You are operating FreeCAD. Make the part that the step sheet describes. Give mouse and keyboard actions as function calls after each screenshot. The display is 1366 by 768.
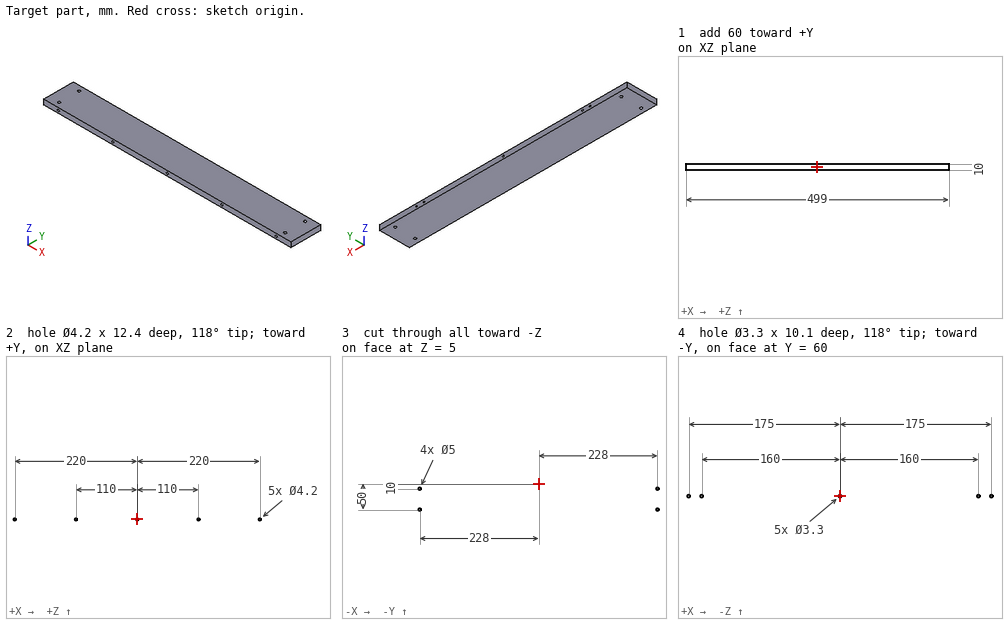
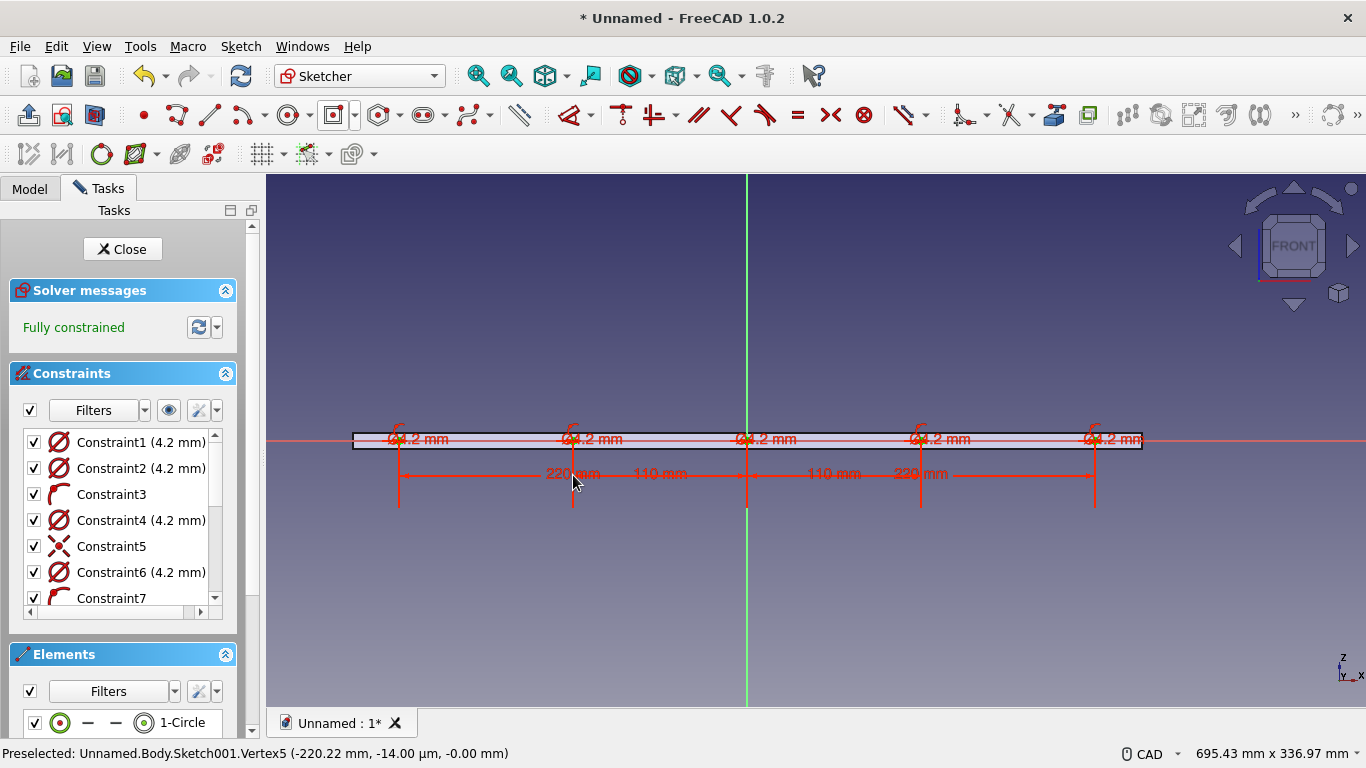
click(123, 249)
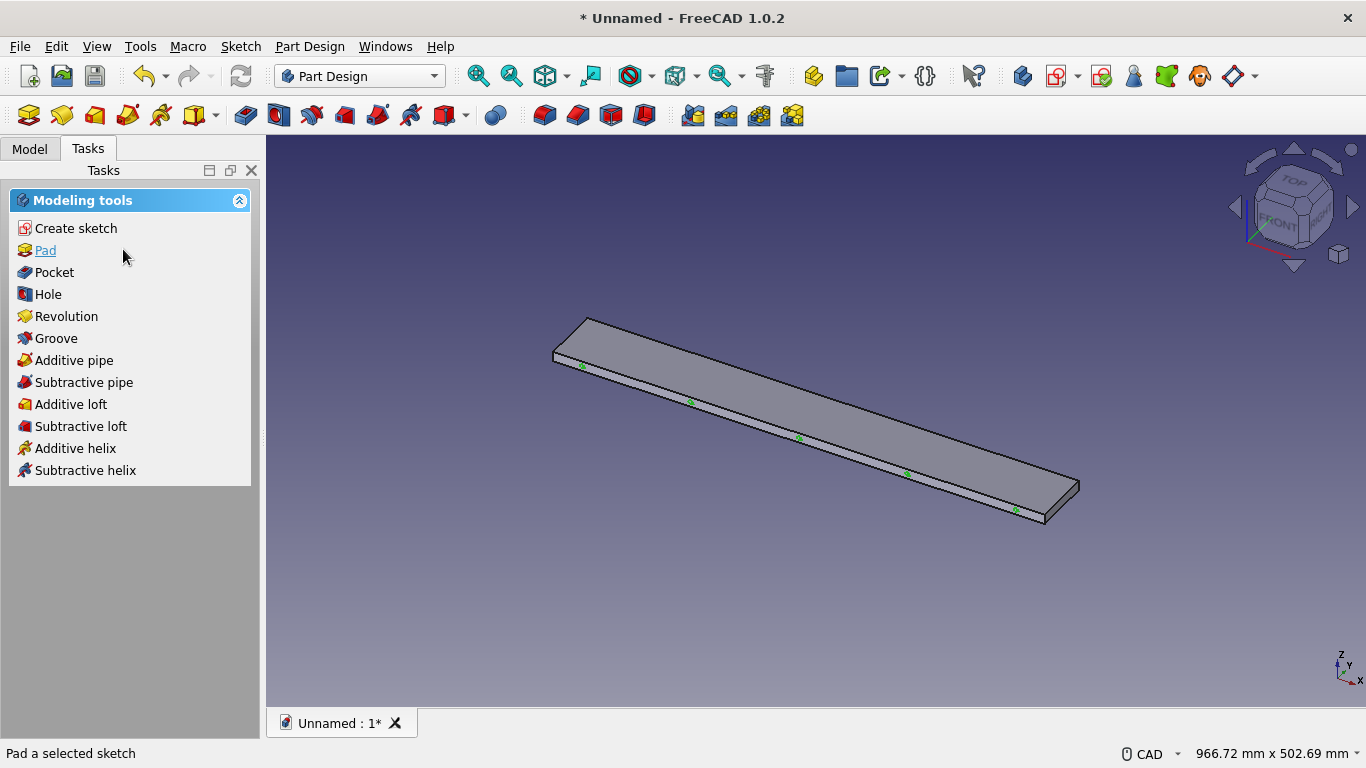
click(279, 116)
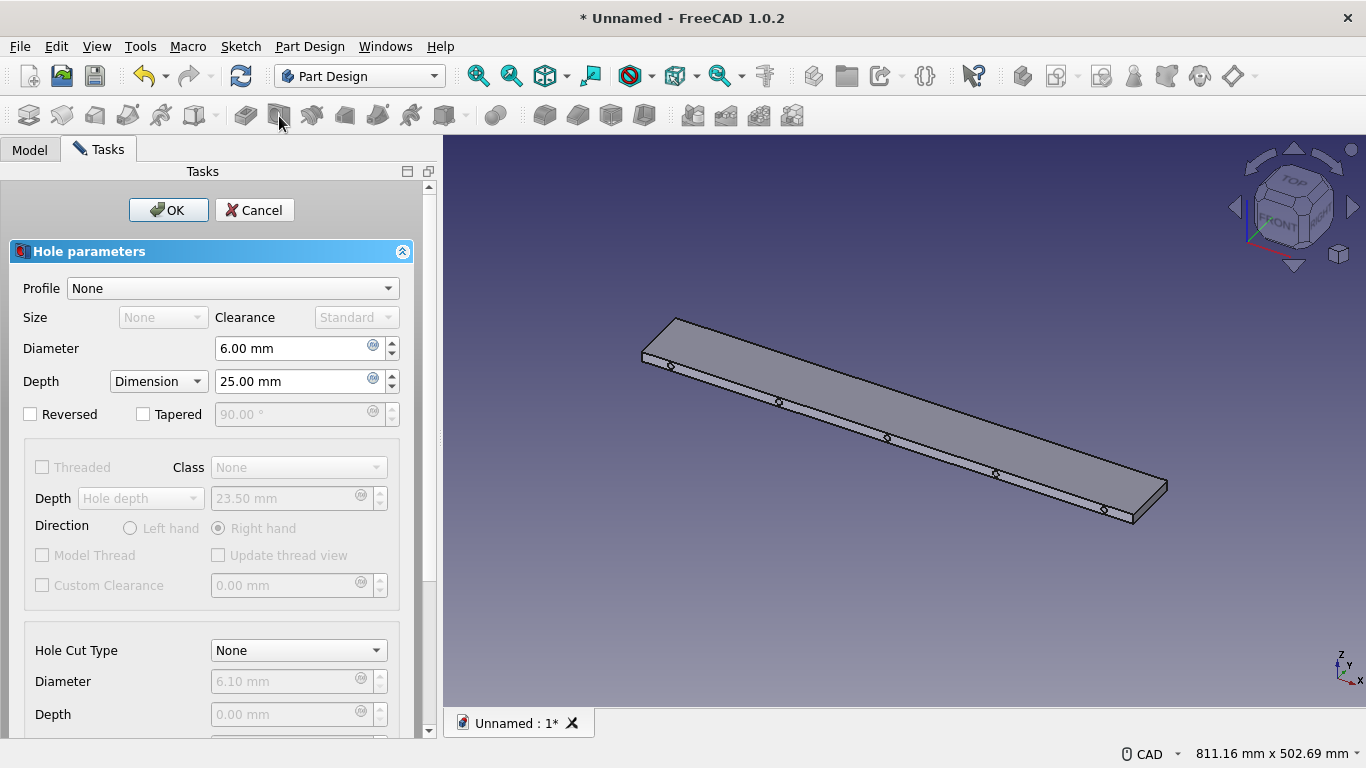
triple_click(300, 348)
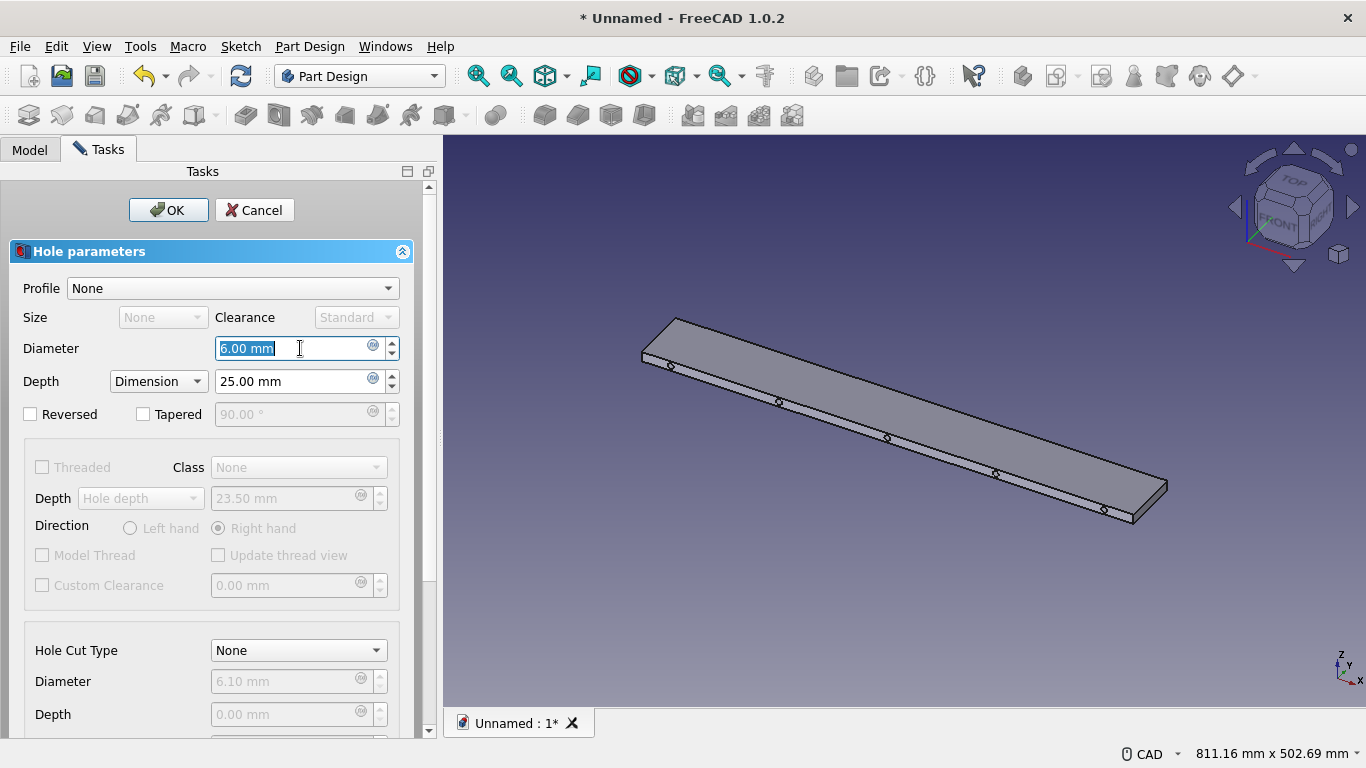
text(4.2)
key(Tab)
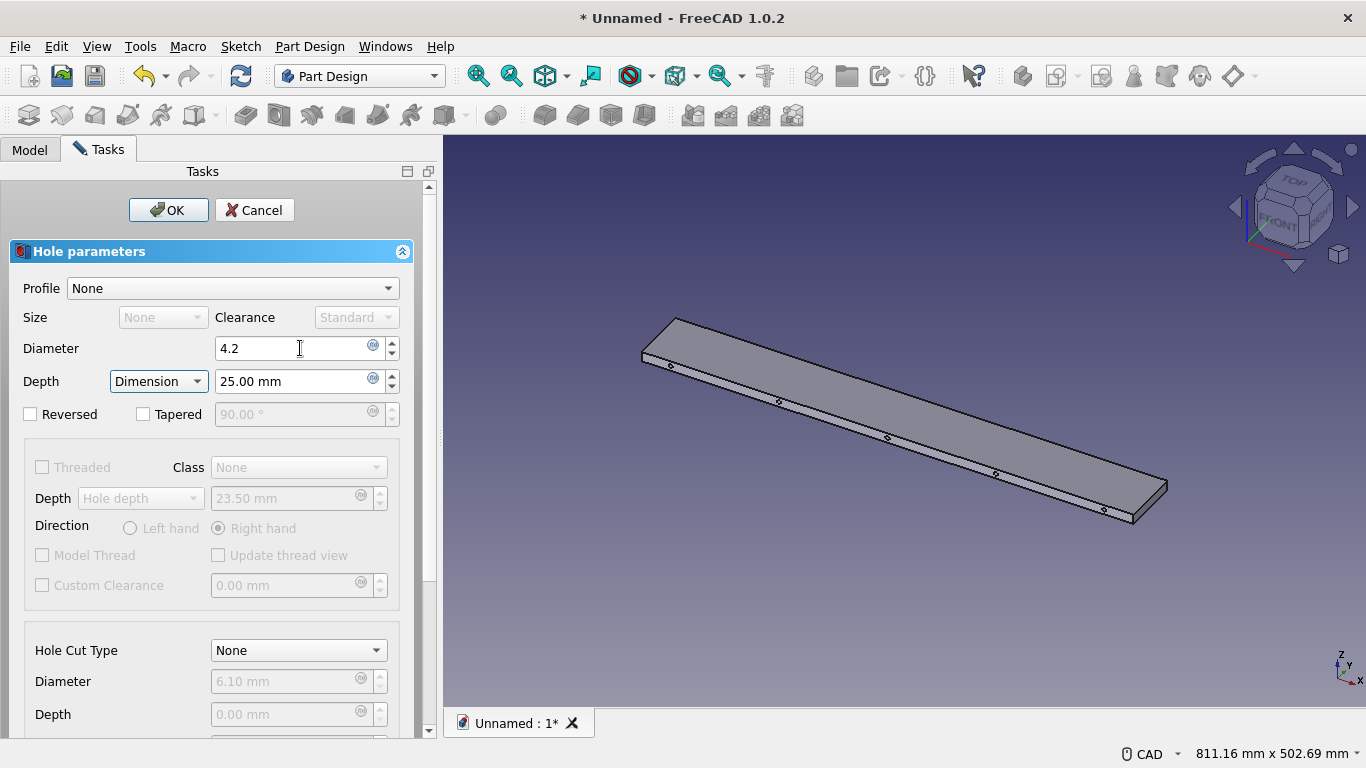
triple_click(300, 382)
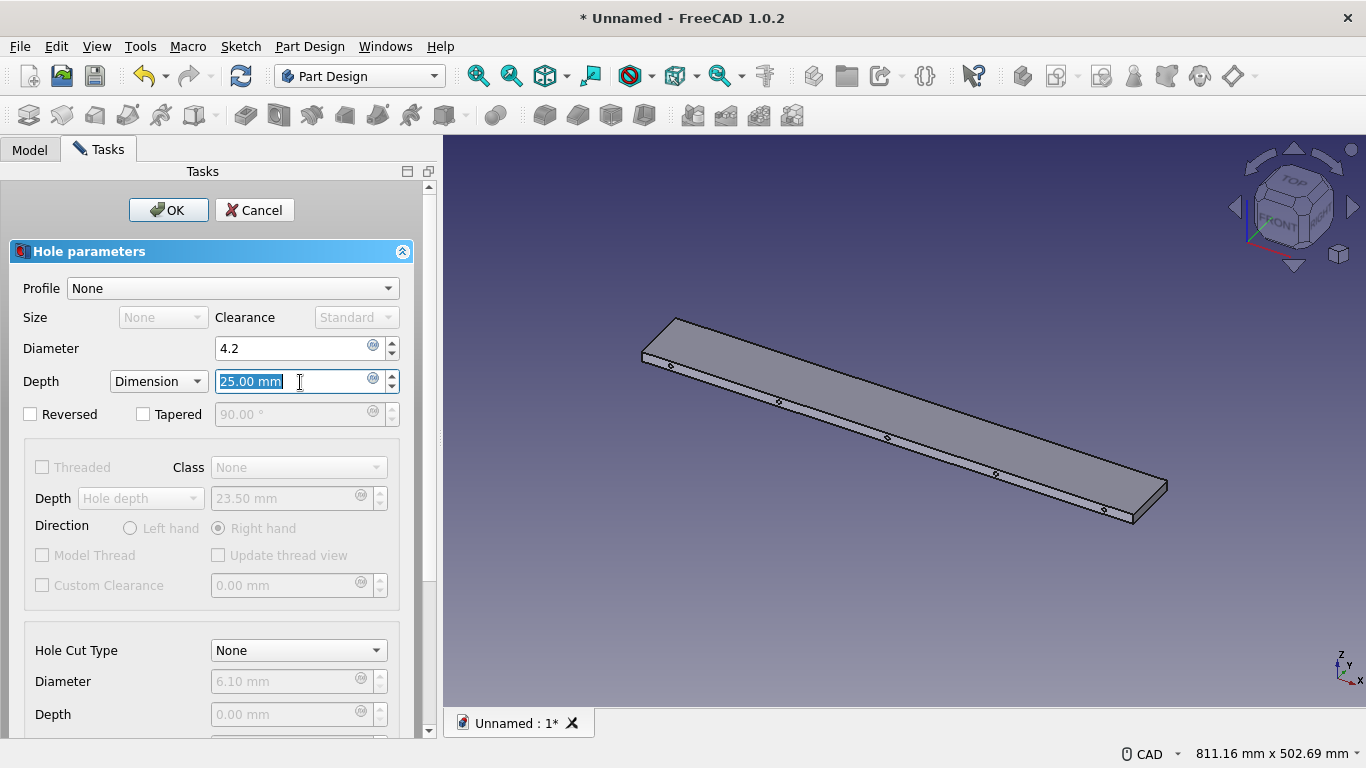
text(12.4)
key(Tab)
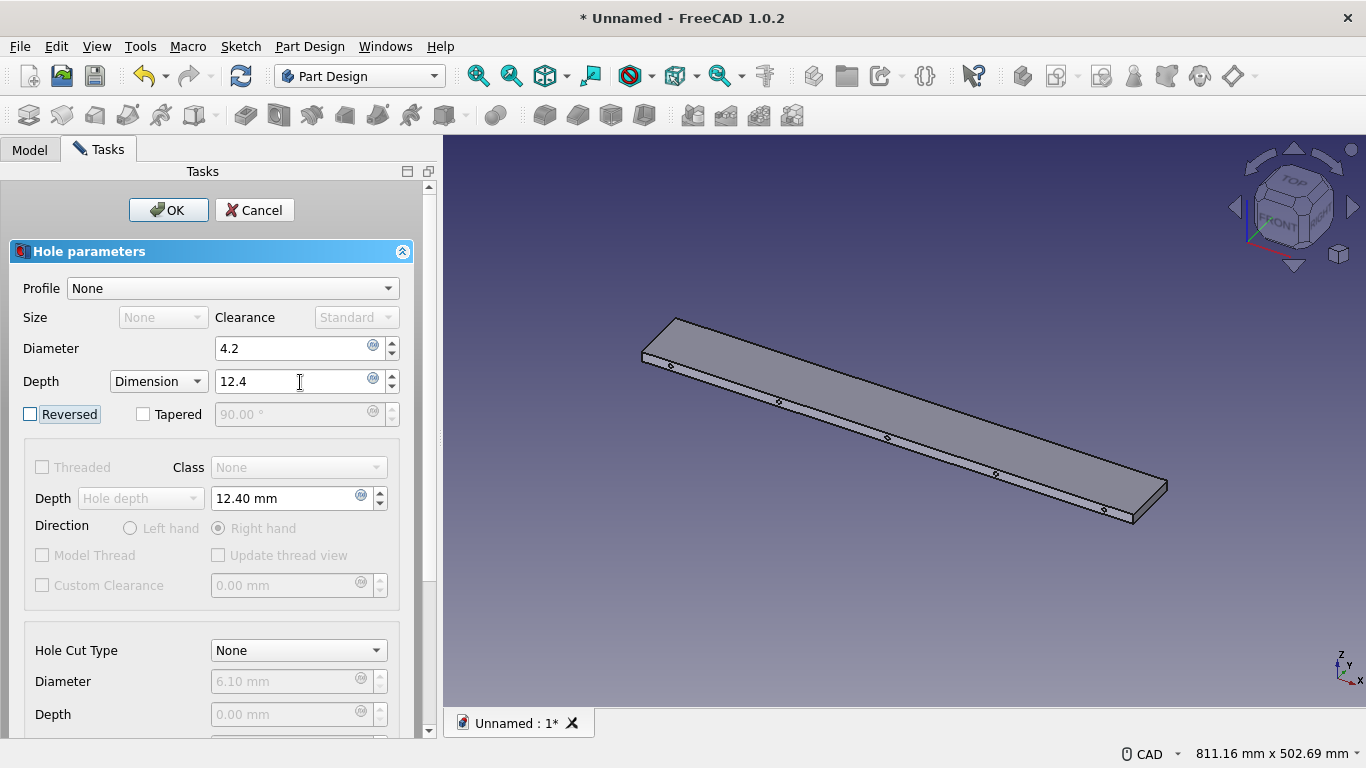
click(169, 210)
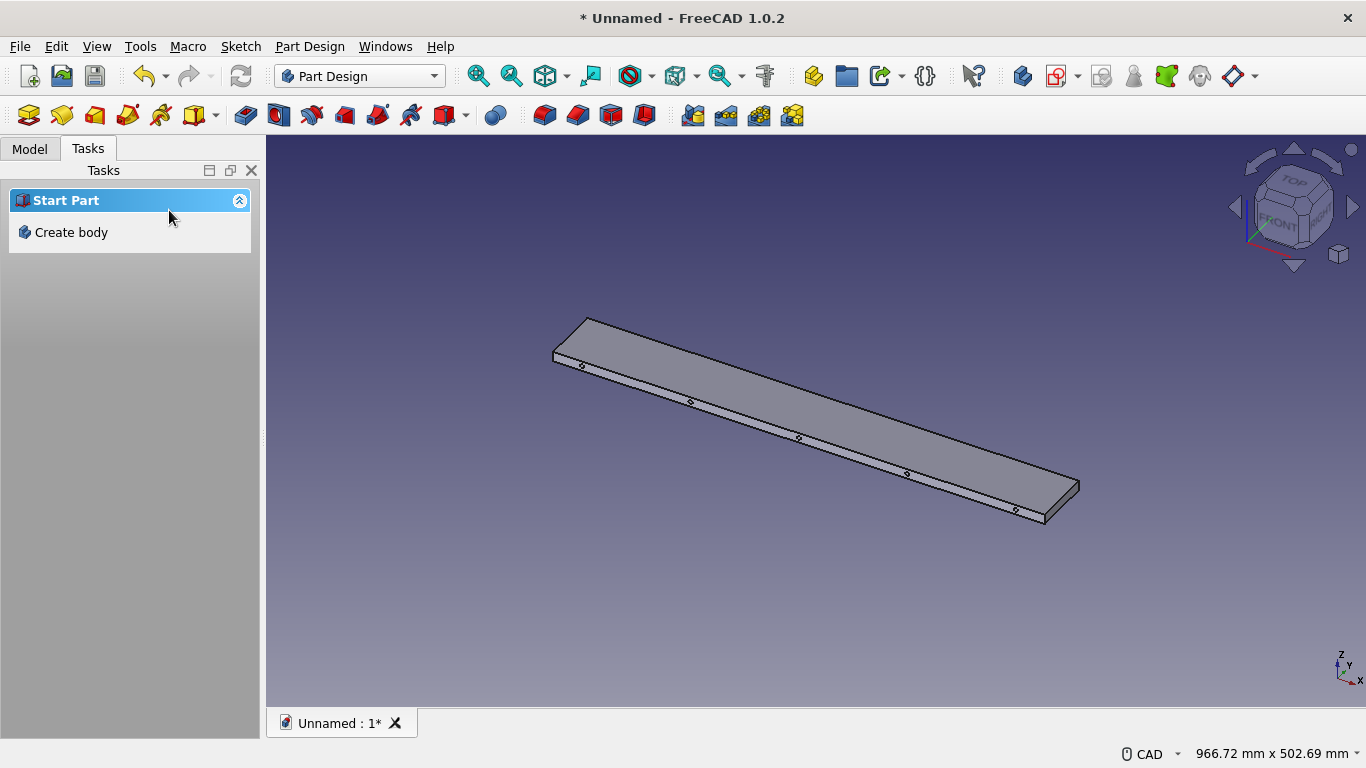
click(1027, 485)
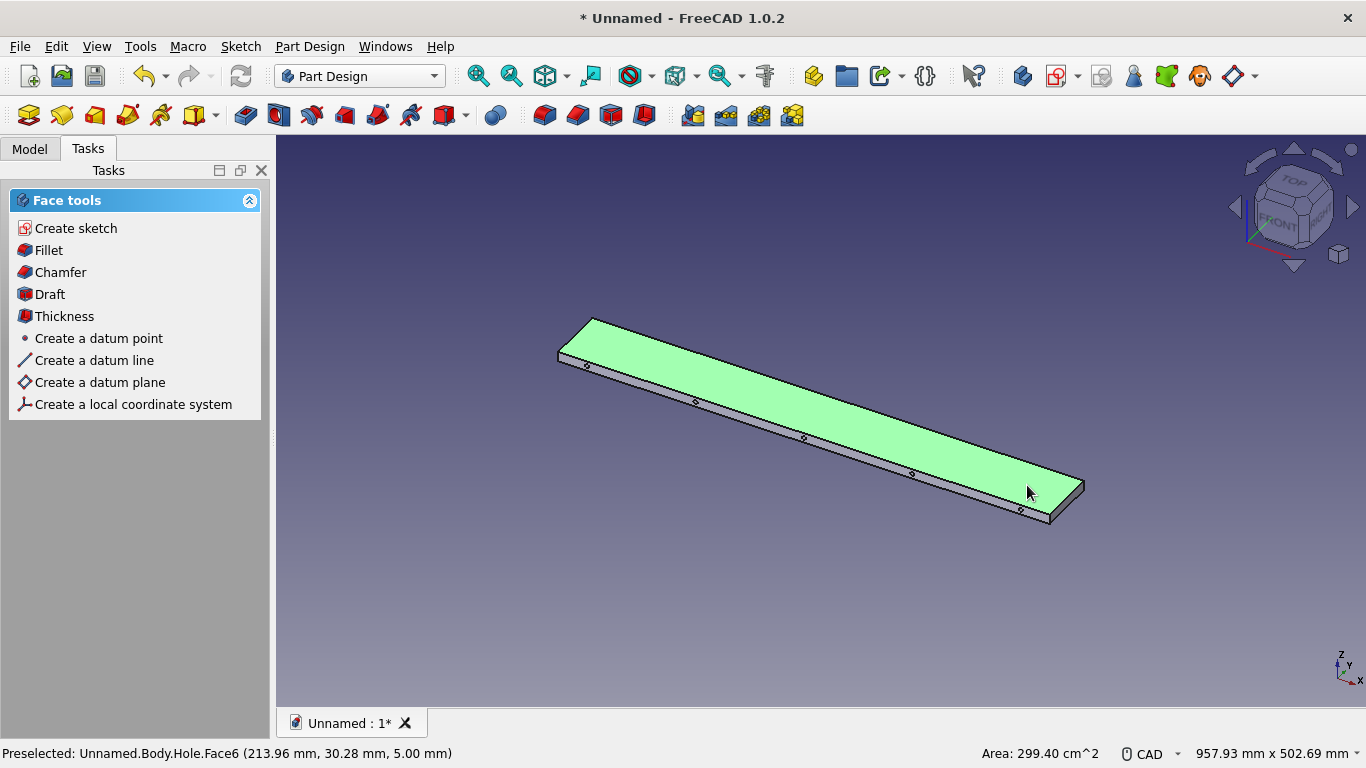
click(1056, 76)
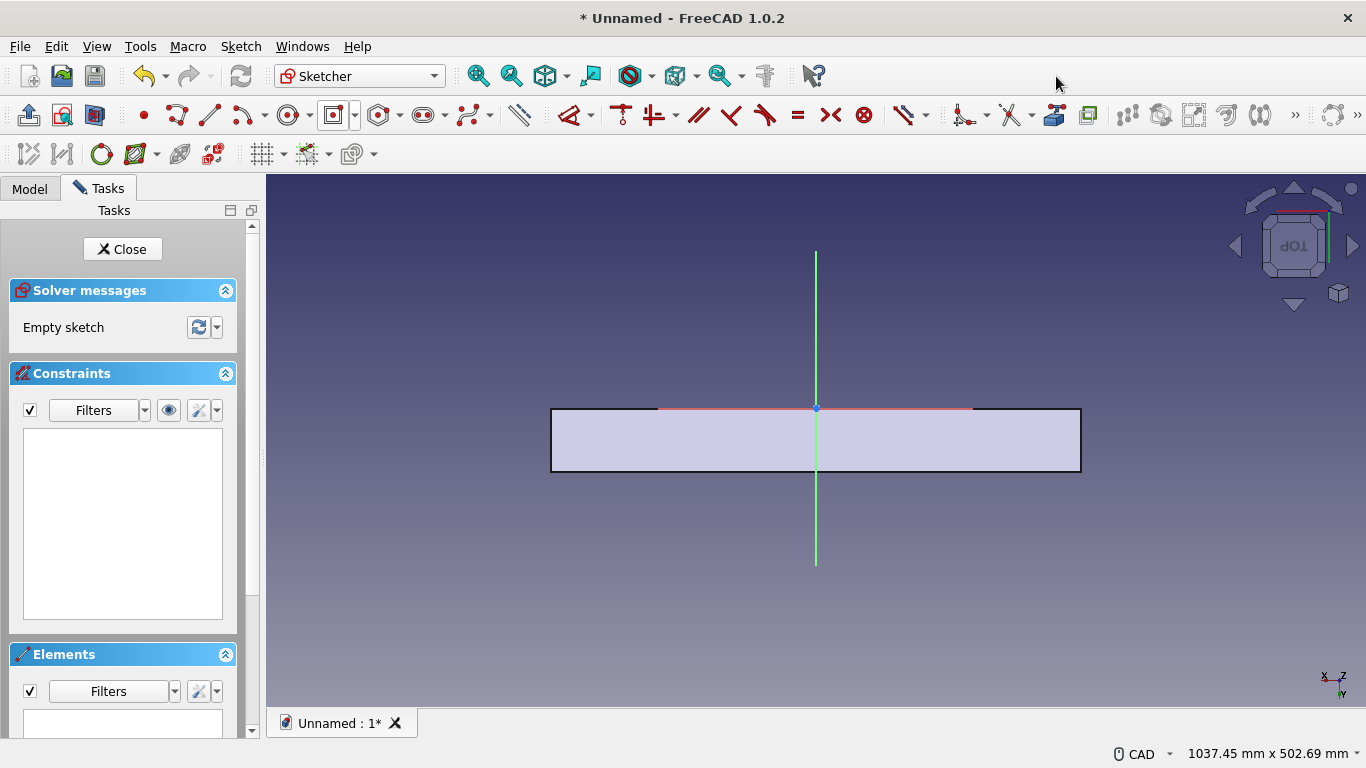
key(g)
key(c)